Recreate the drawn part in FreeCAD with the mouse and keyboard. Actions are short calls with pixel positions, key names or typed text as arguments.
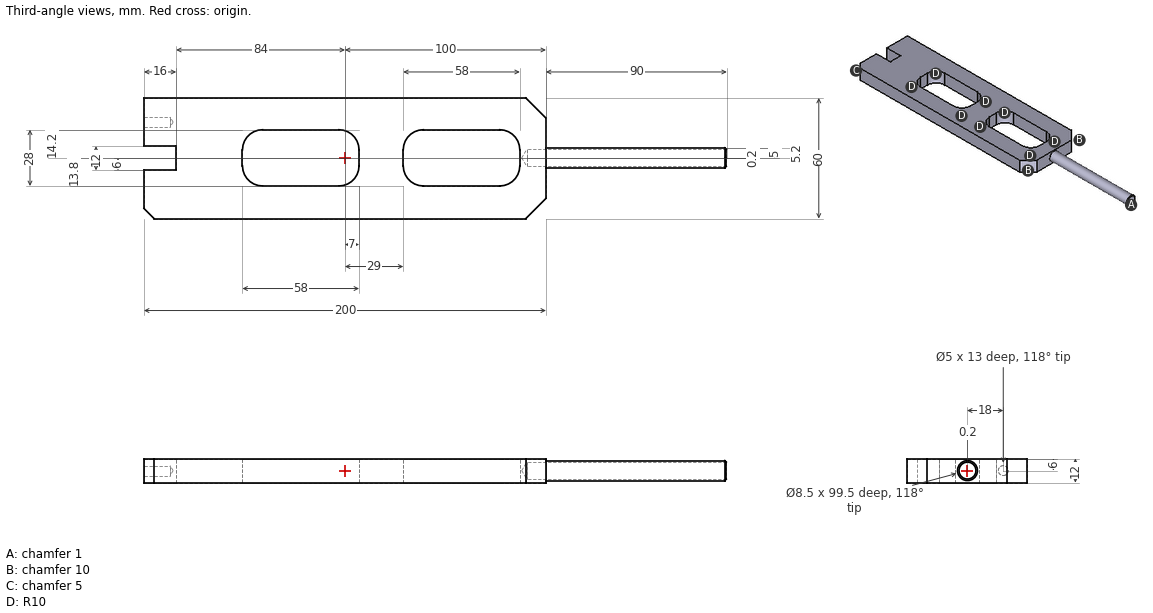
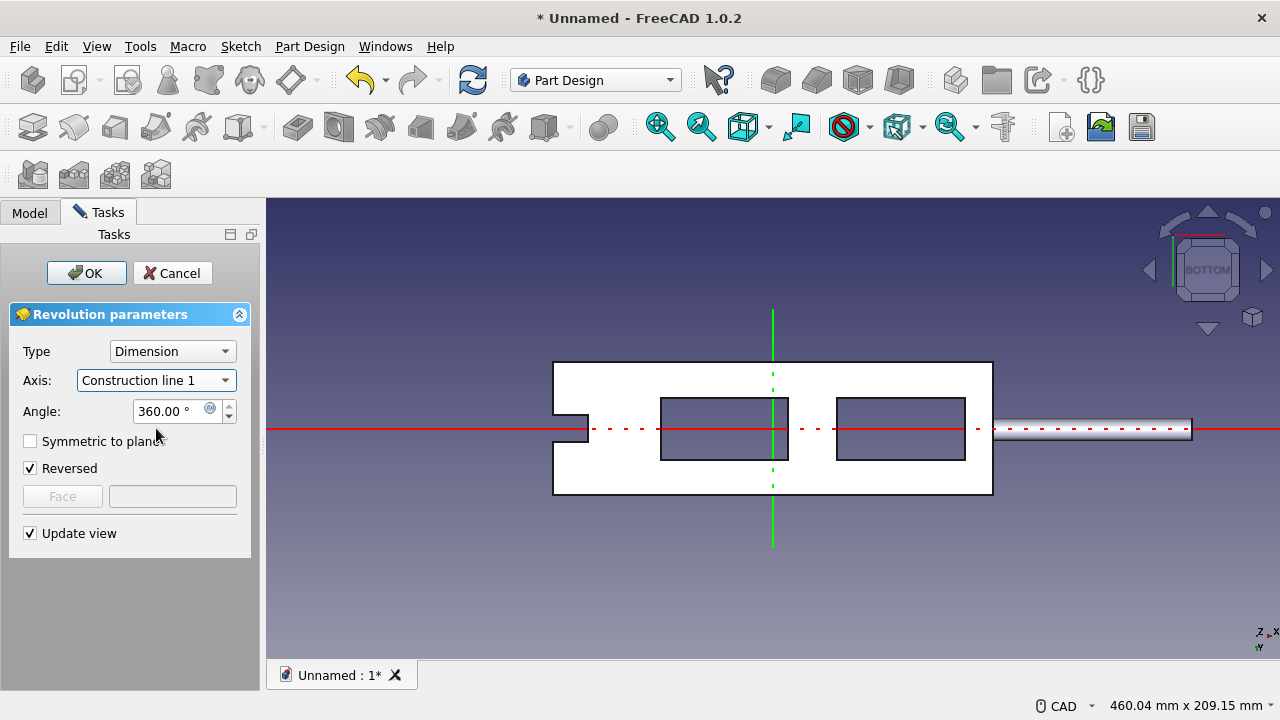
click(87, 273)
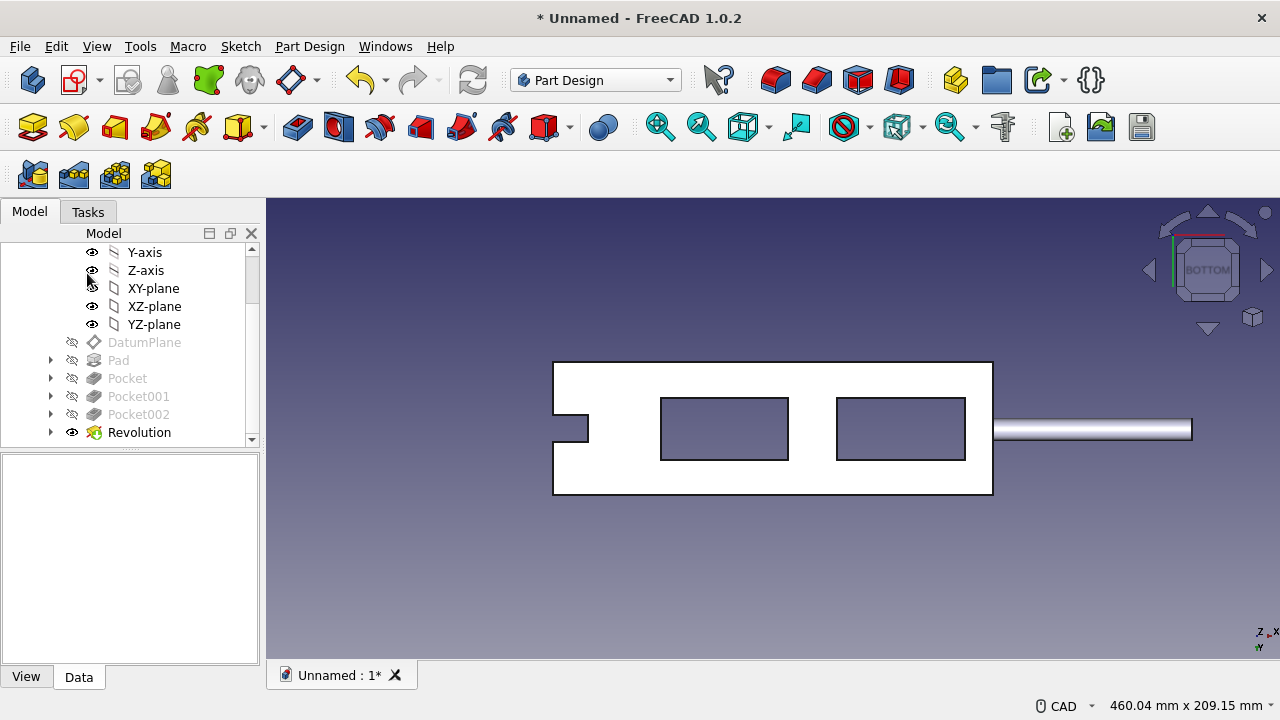
key(6)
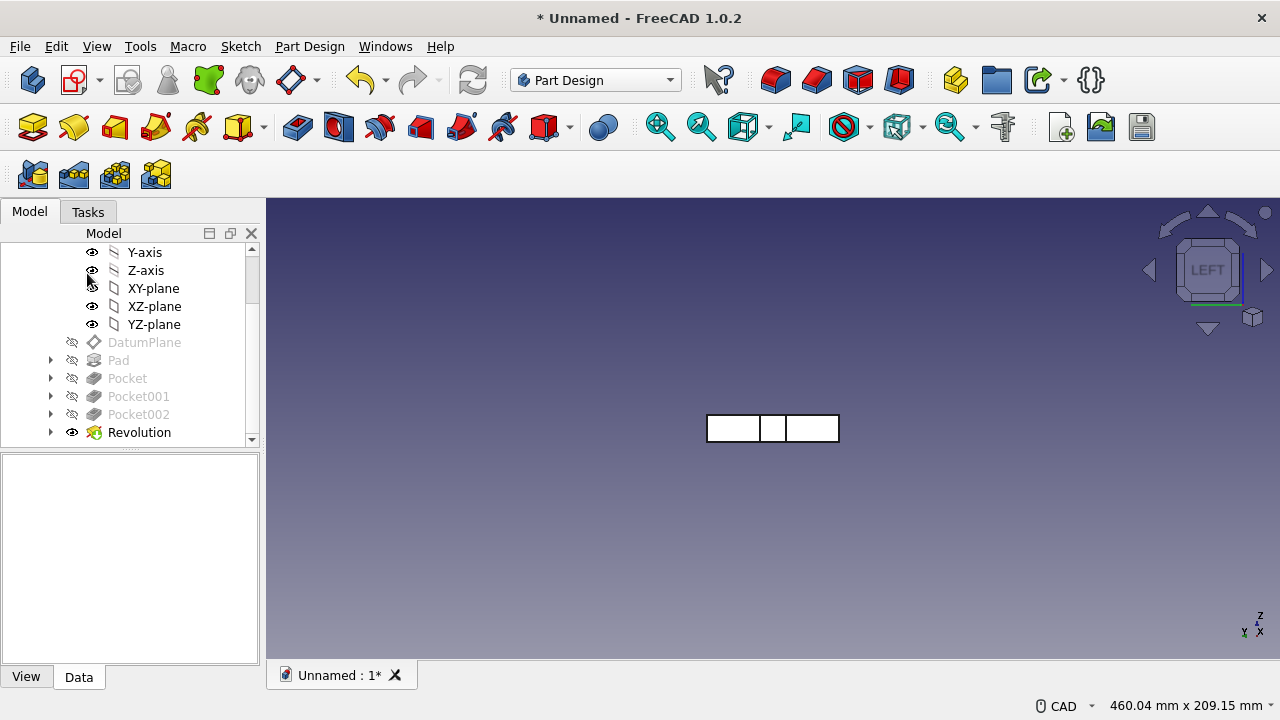
key(v)
key(f)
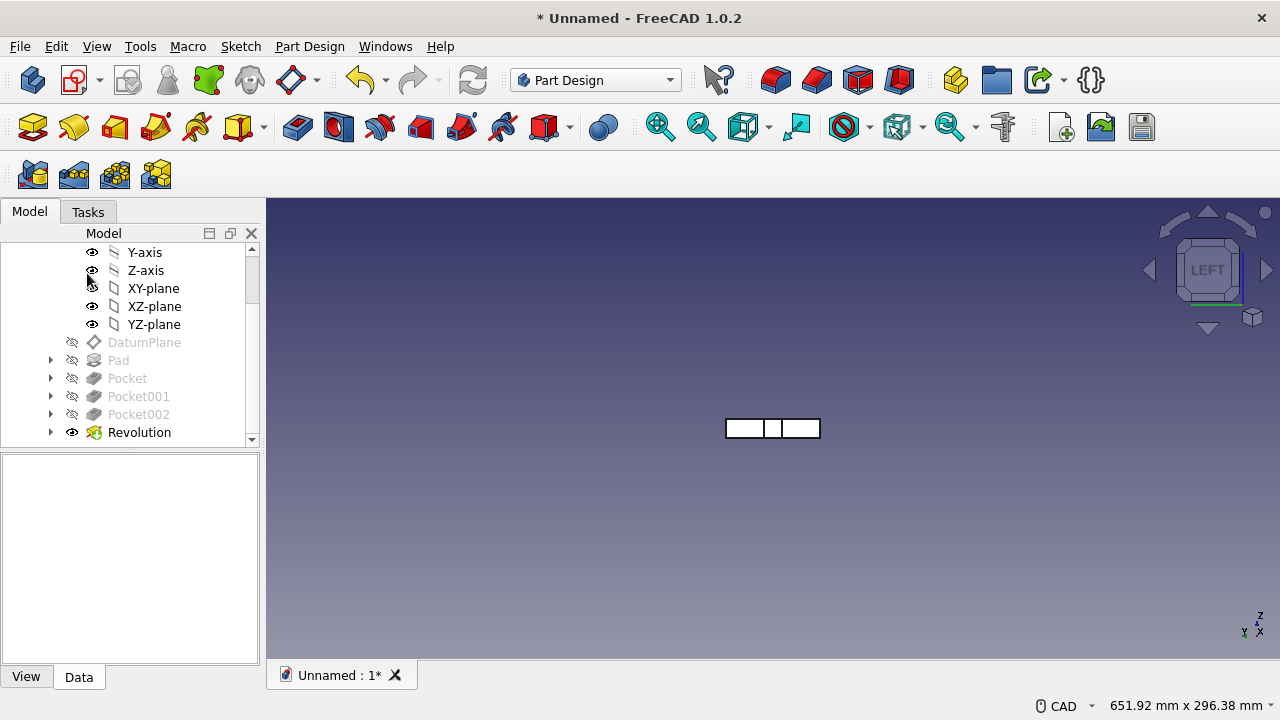
click(796, 427)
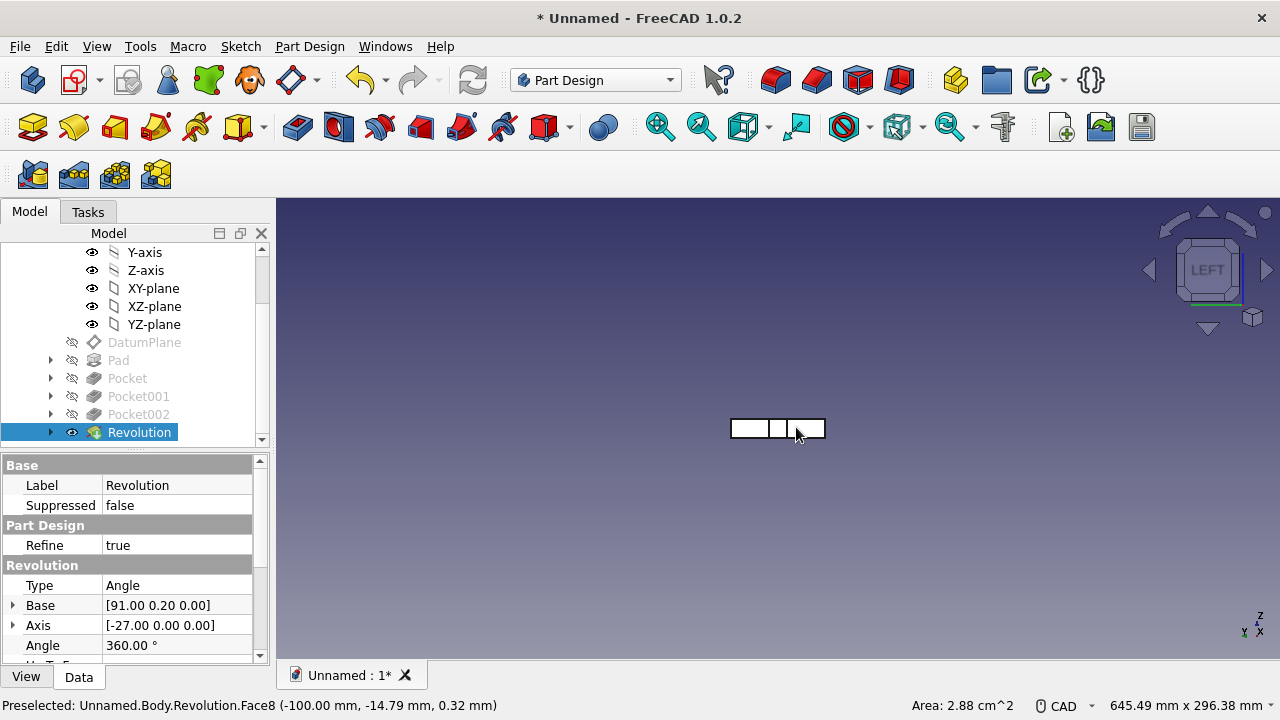
click(74, 80)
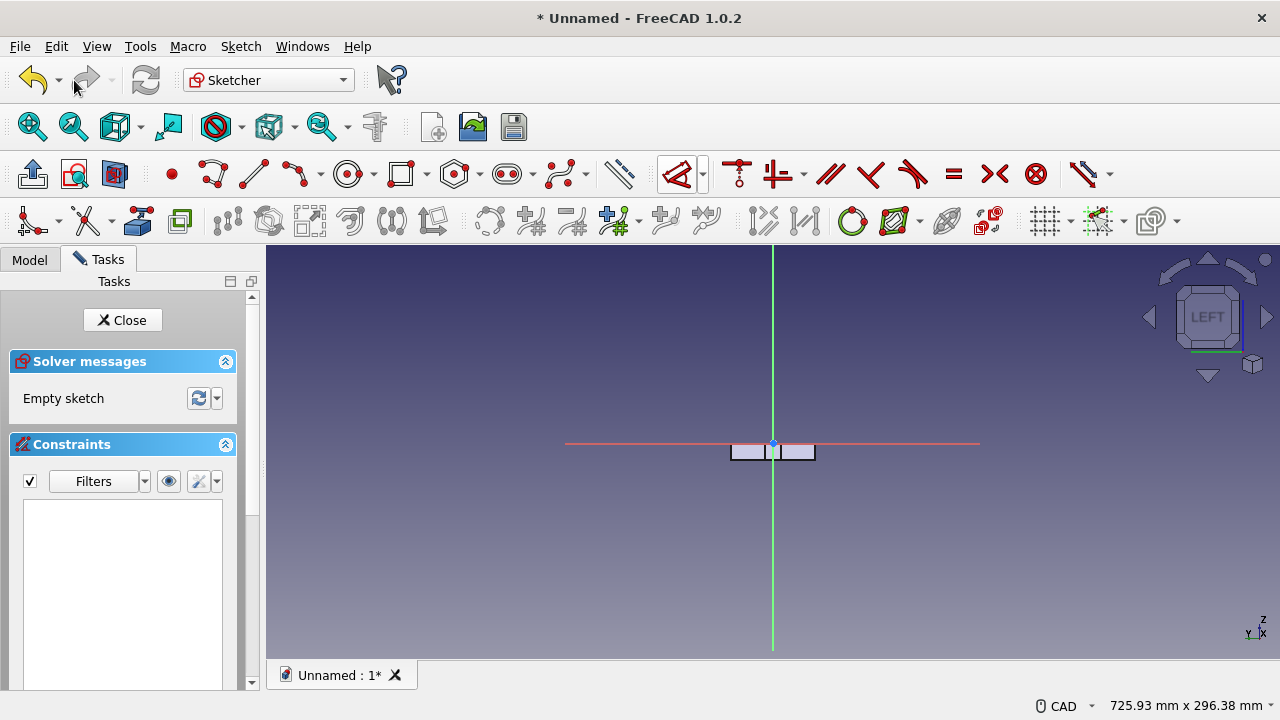
scroll(750, 452, up, 15)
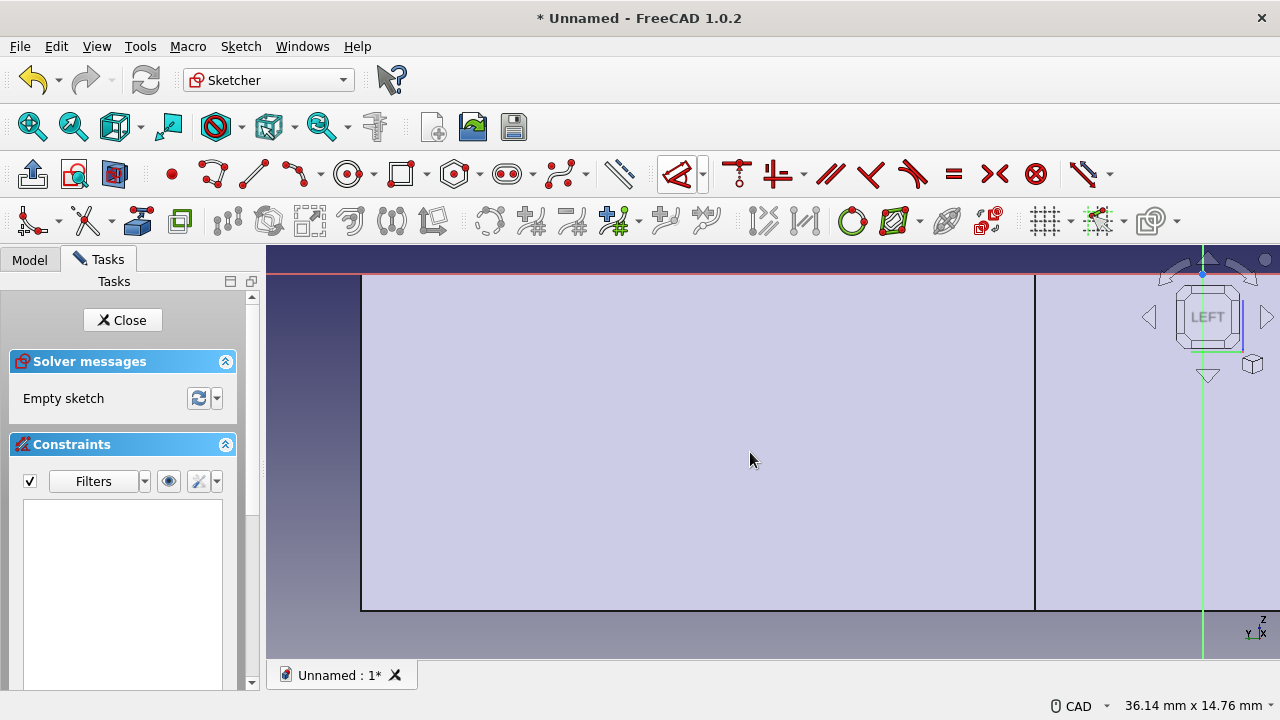
scroll(690, 431, up, 3)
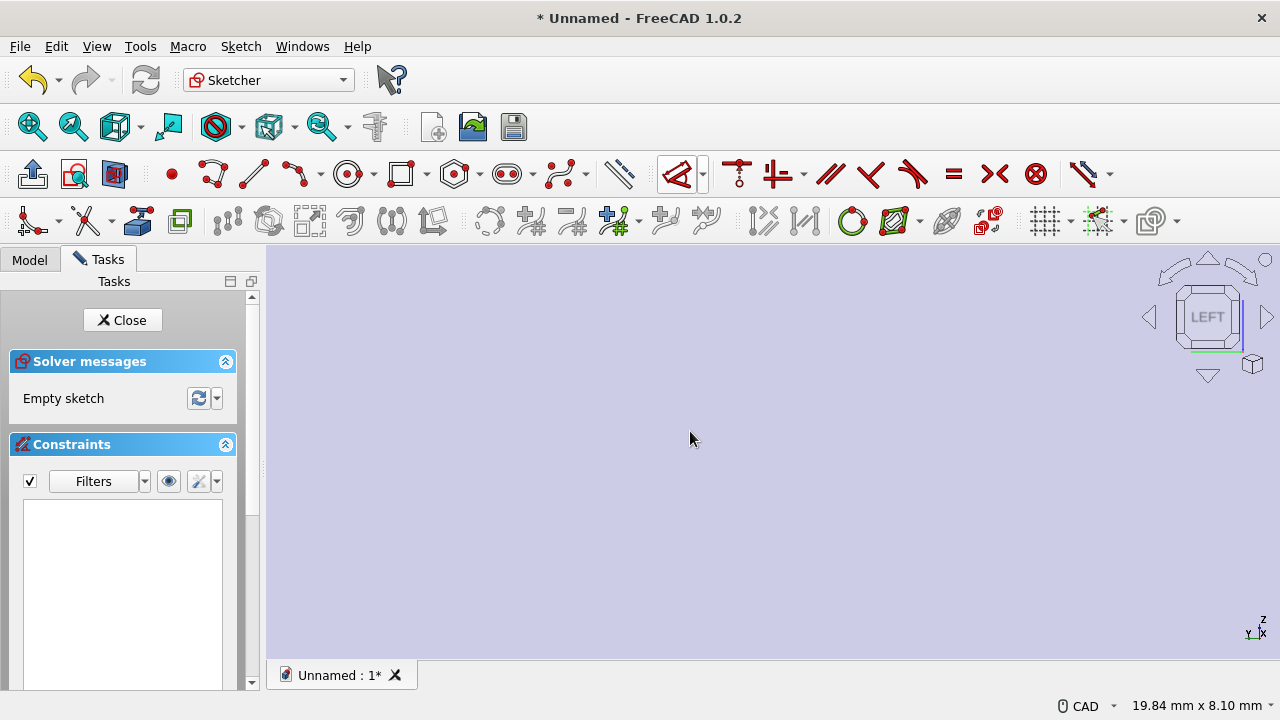
key(g)
key(c)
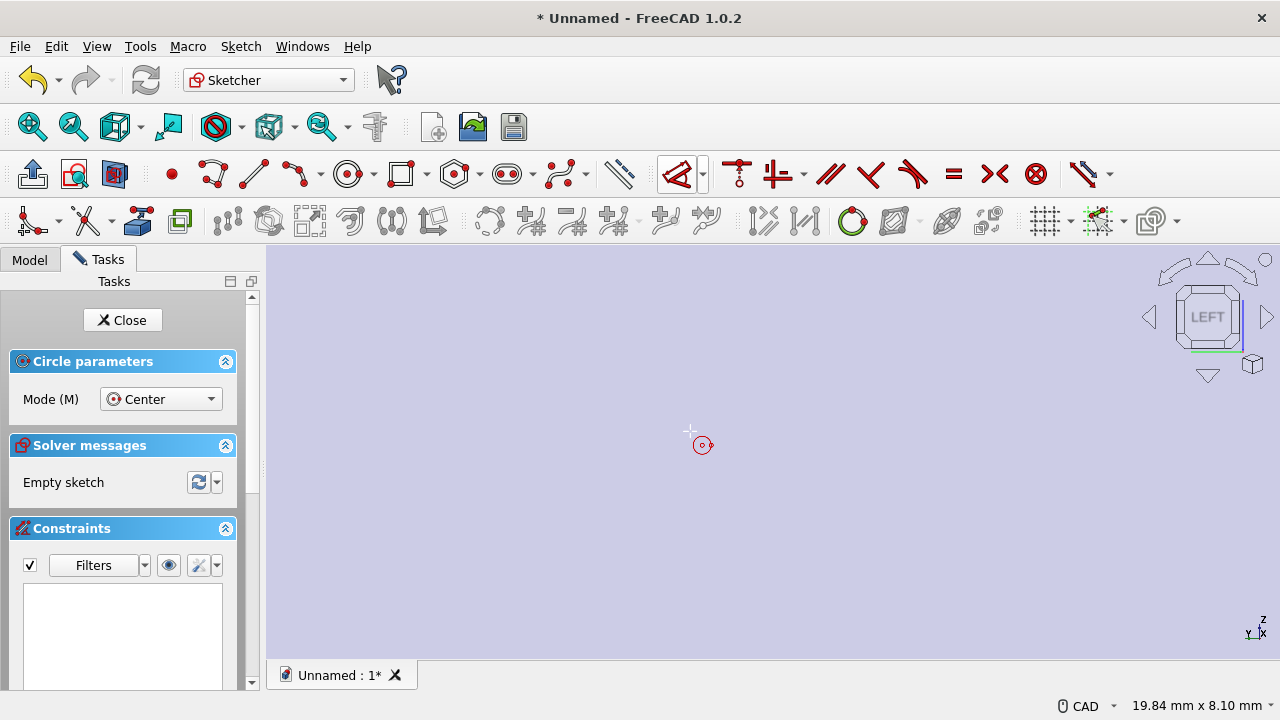
click(704, 451)
move(794, 361)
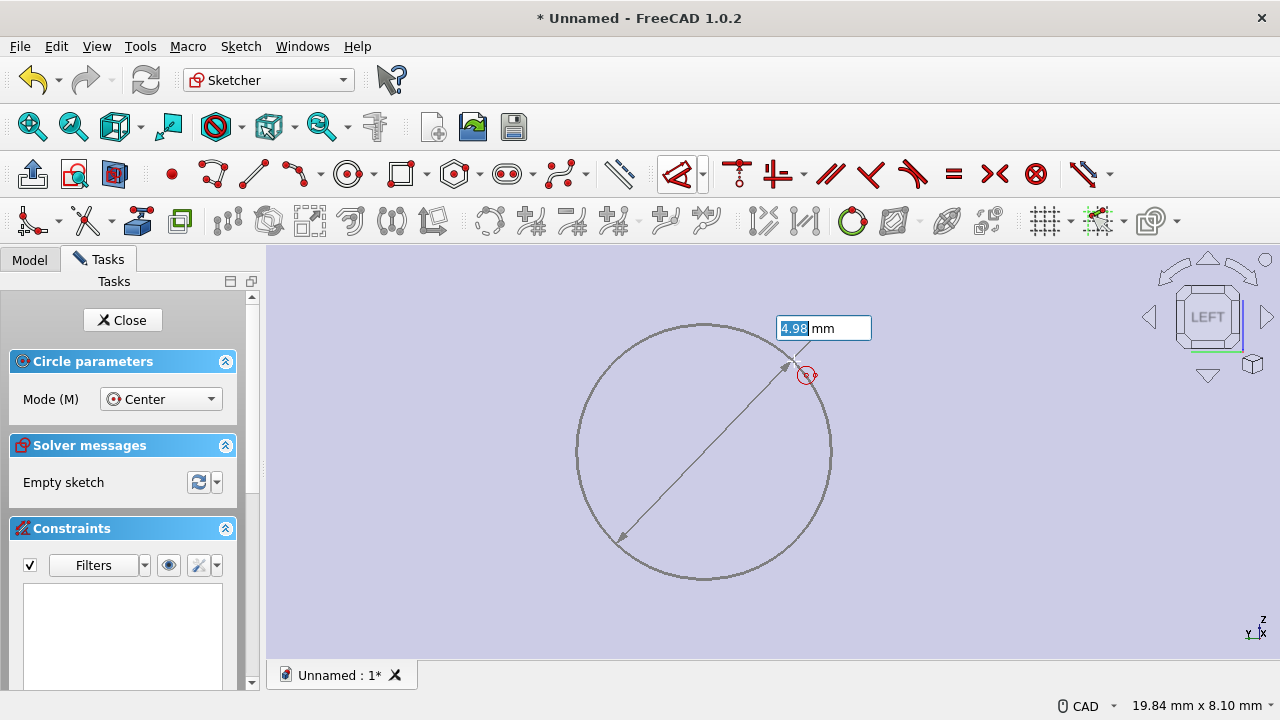
text(5)
key(Return)
key(Escape)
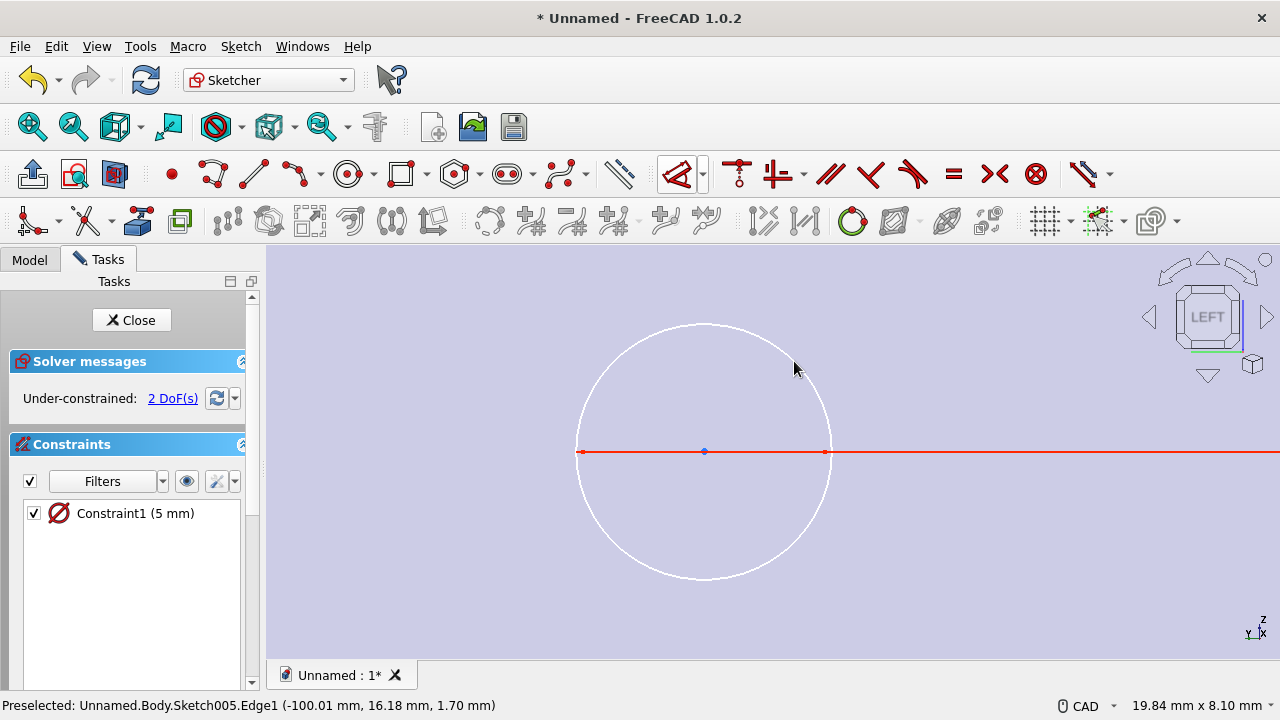
click(704, 452)